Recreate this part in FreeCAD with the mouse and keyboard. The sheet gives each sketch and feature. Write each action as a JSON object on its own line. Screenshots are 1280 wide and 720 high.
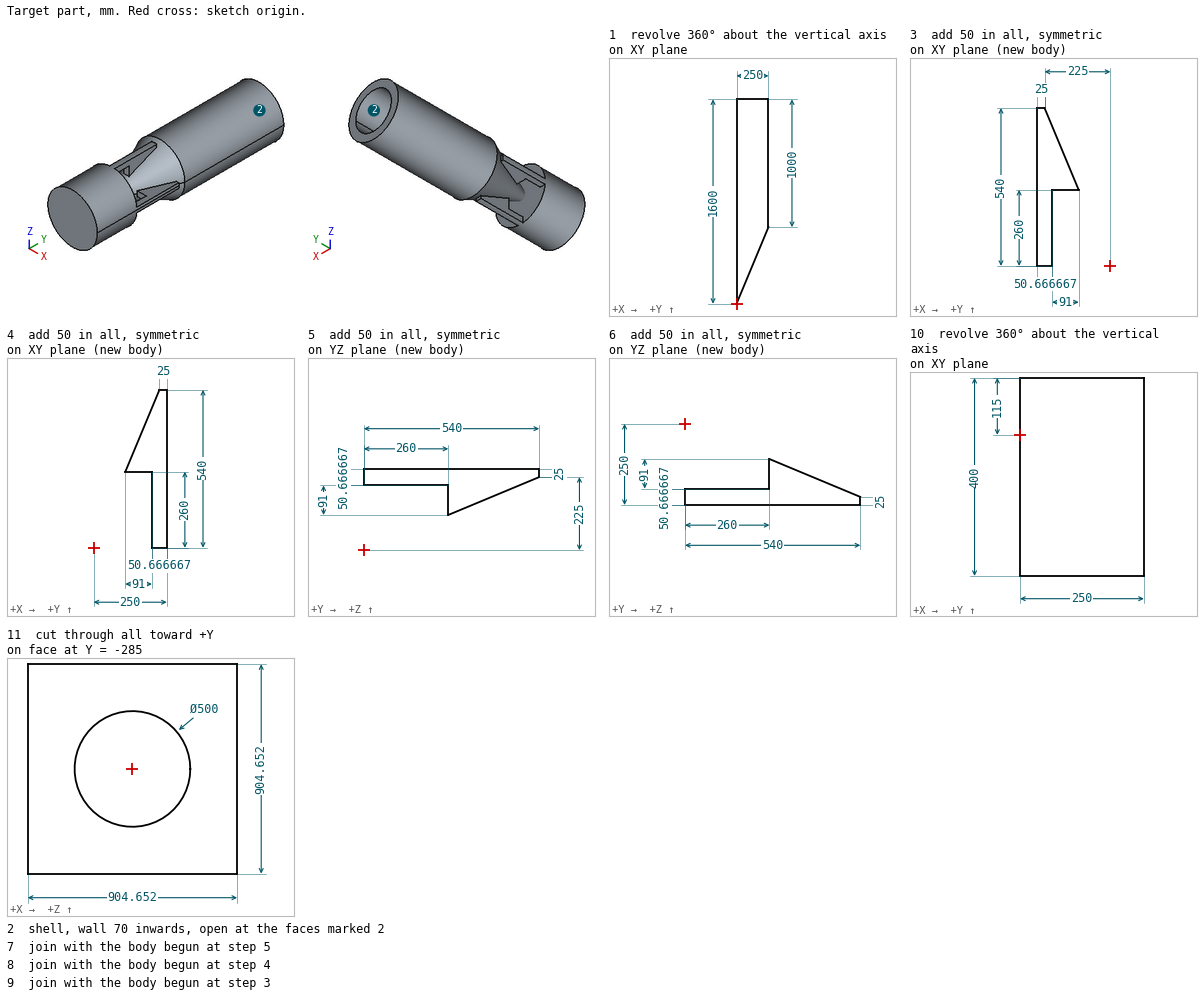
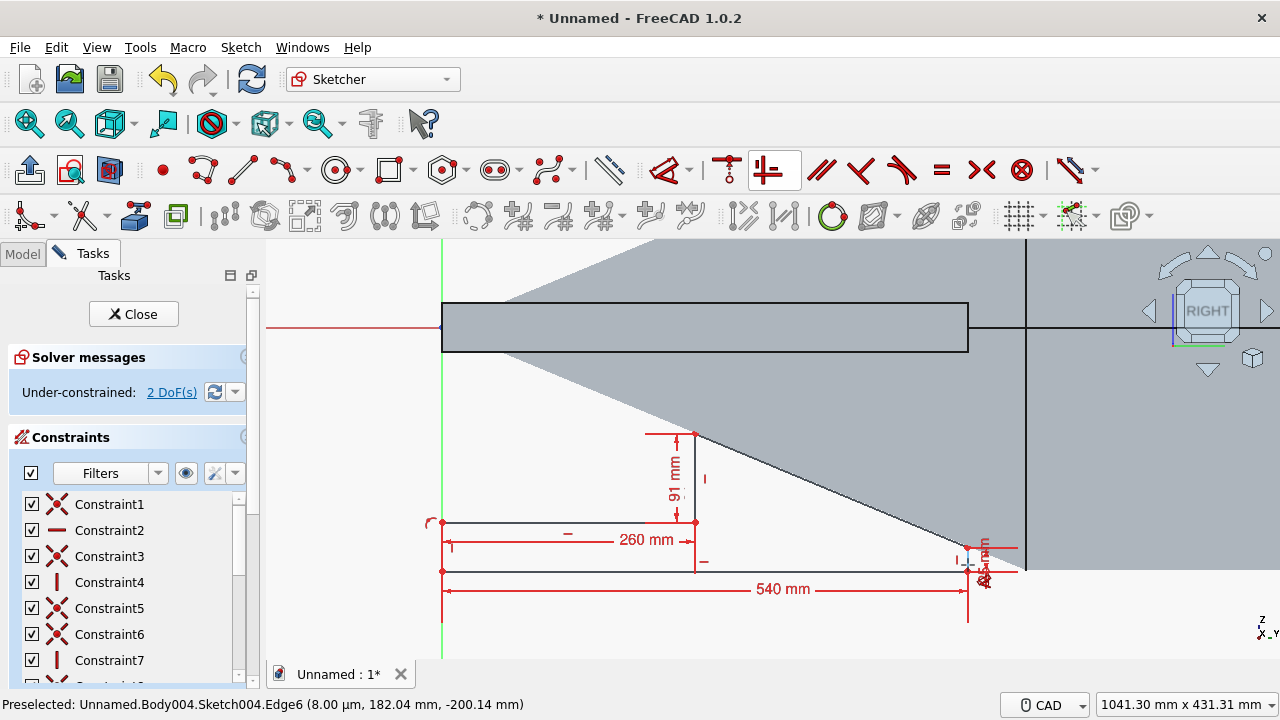
{"action": "left_click", "coordinate": [442, 572]}
{"action": "left_click", "coordinate": [408, 450]}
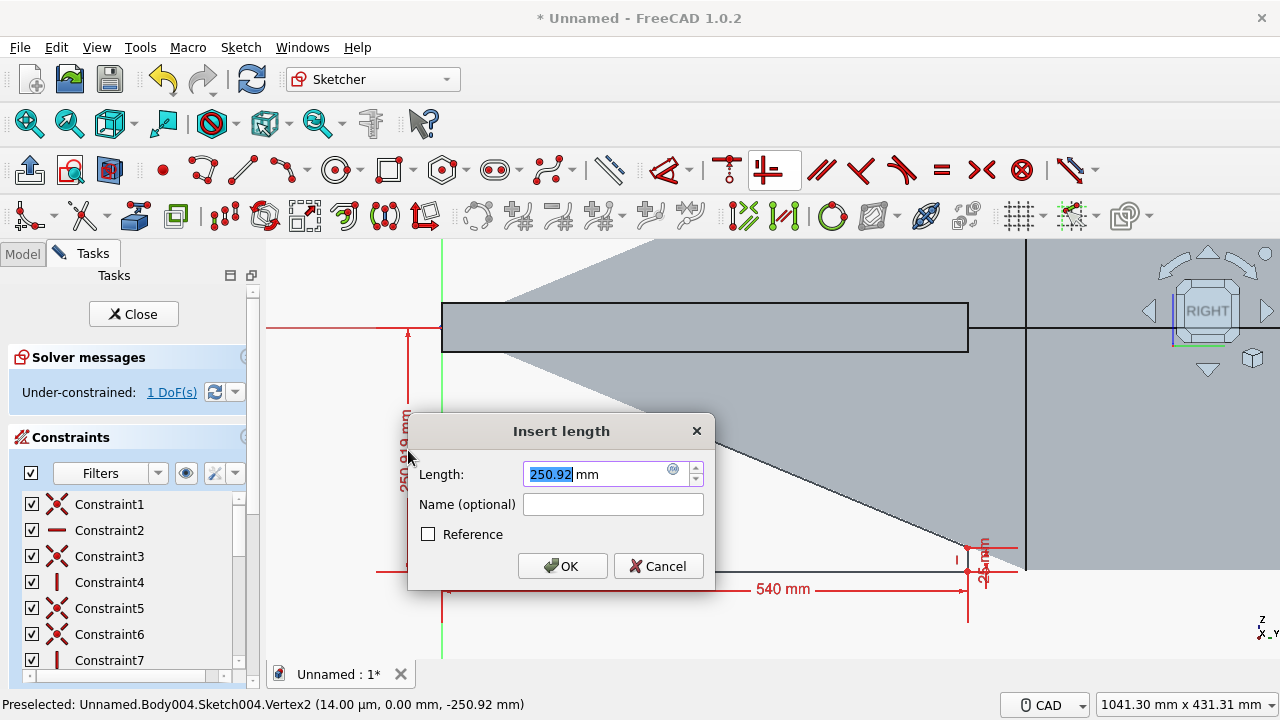
{"action": "type", "text": "250"}
{"action": "key", "text": "Return"}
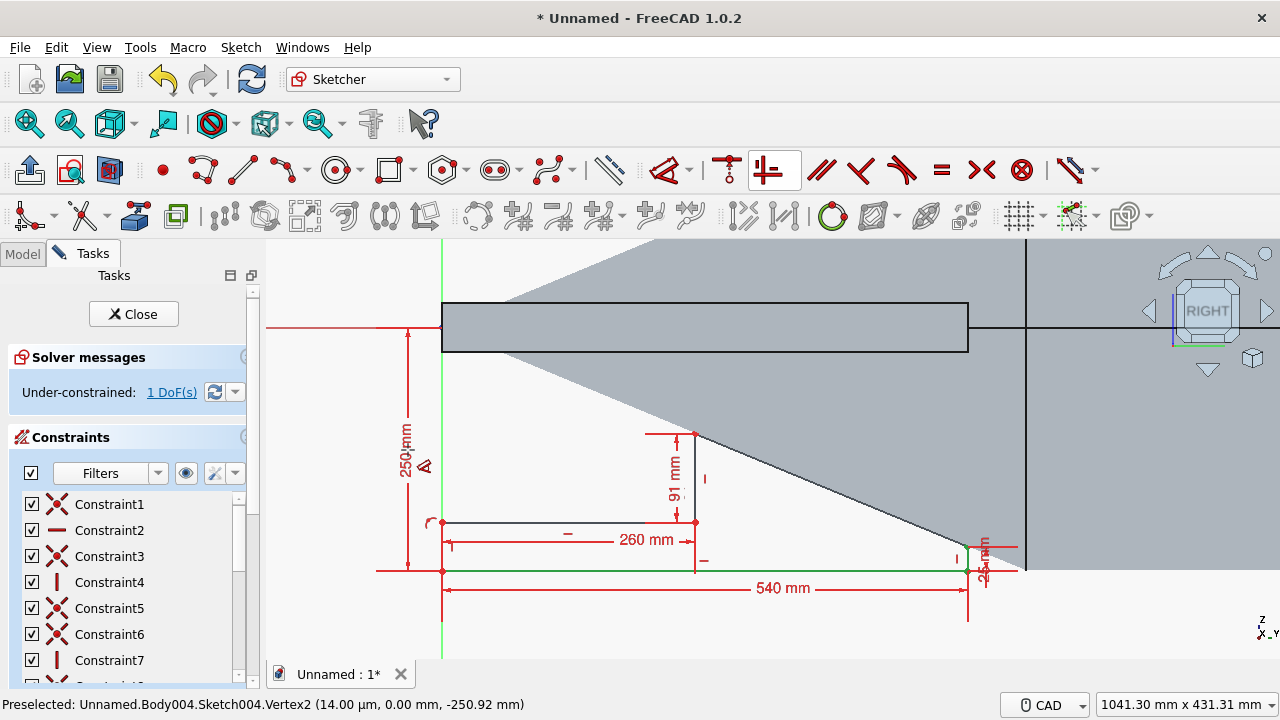
{"action": "left_click", "coordinate": [442, 537]}
{"action": "left_click", "coordinate": [408, 547]}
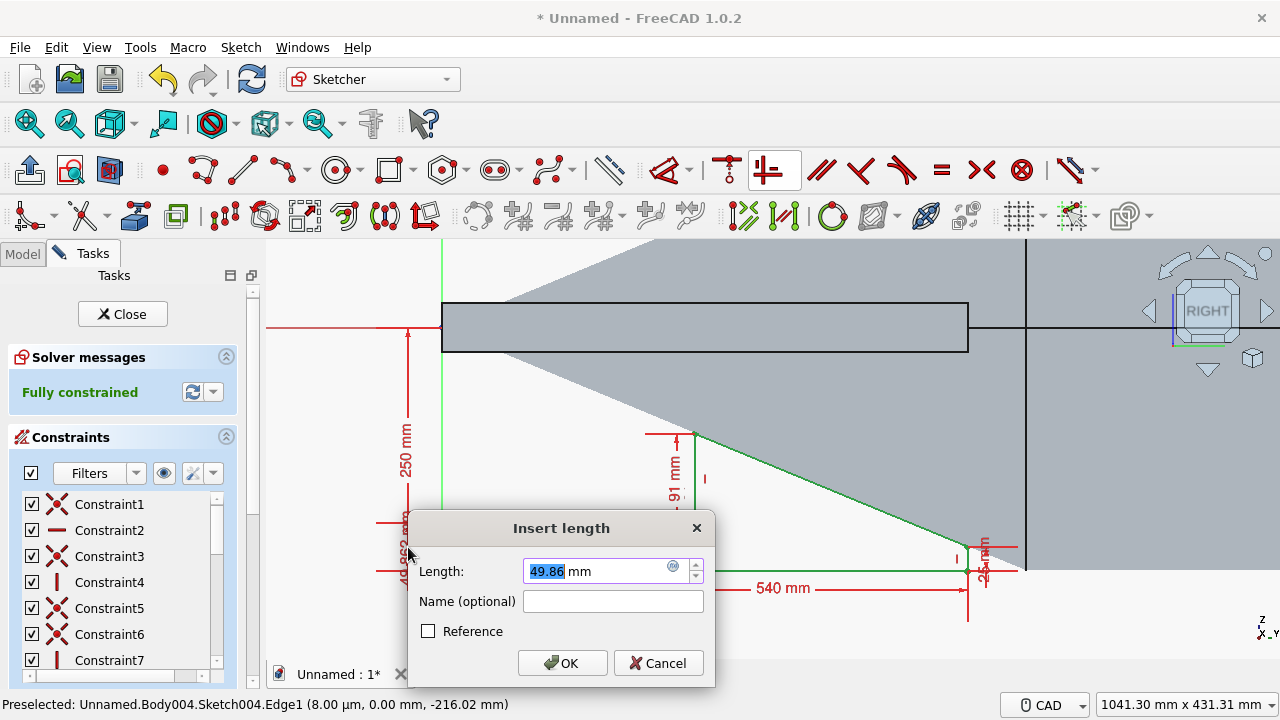
{"action": "type", "text": "50.666667"}
{"action": "key", "text": "Return"}
{"action": "key", "text": "Escape"}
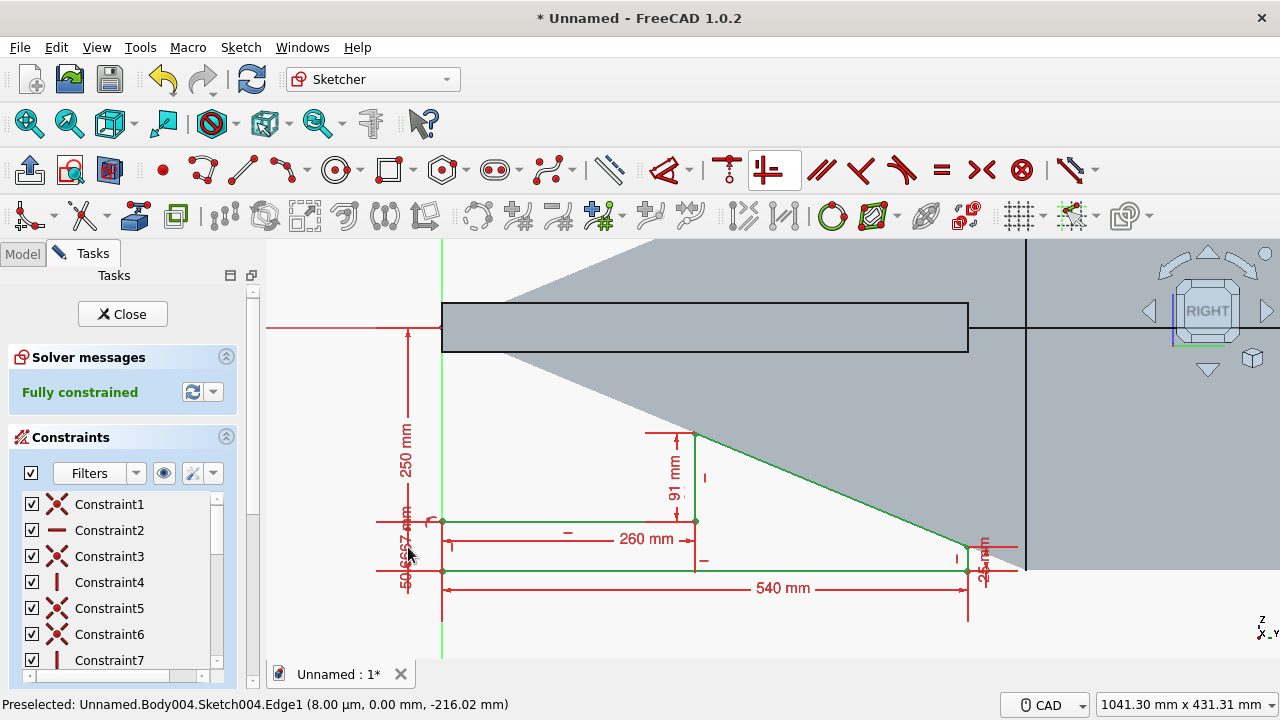
{"action": "left_click", "coordinate": [123, 314]}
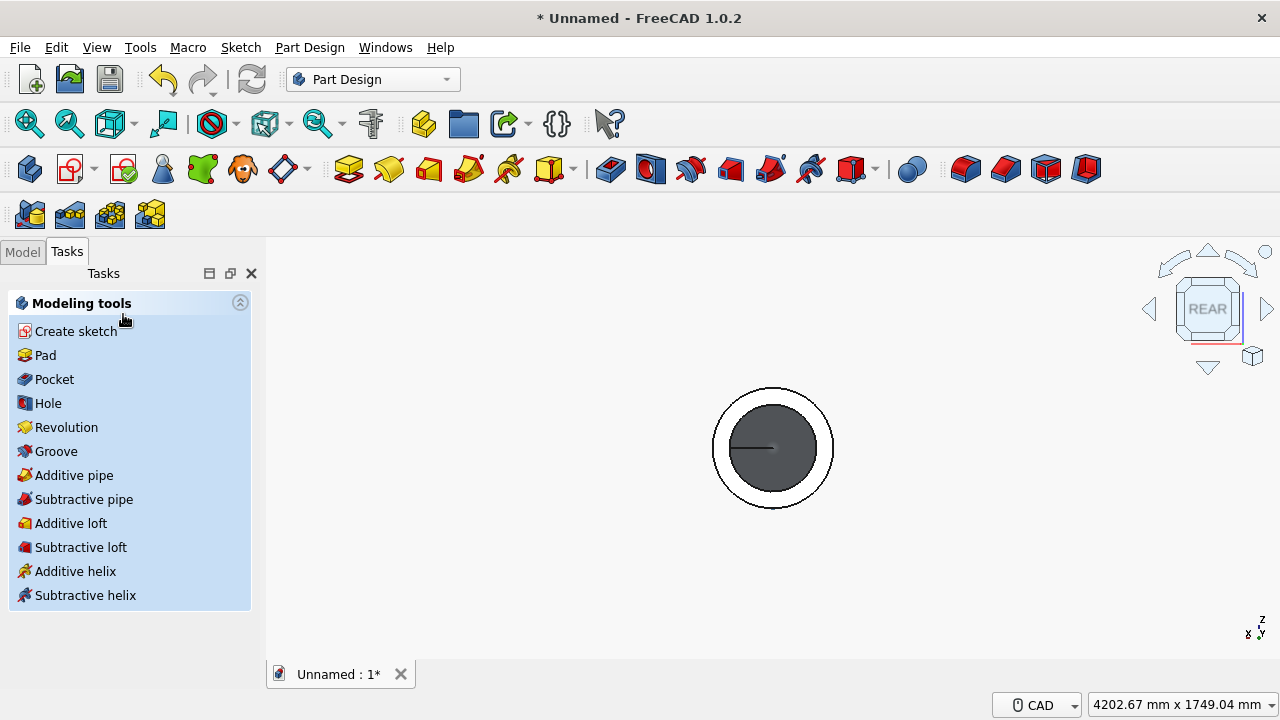
{"action": "left_click", "coordinate": [350, 170]}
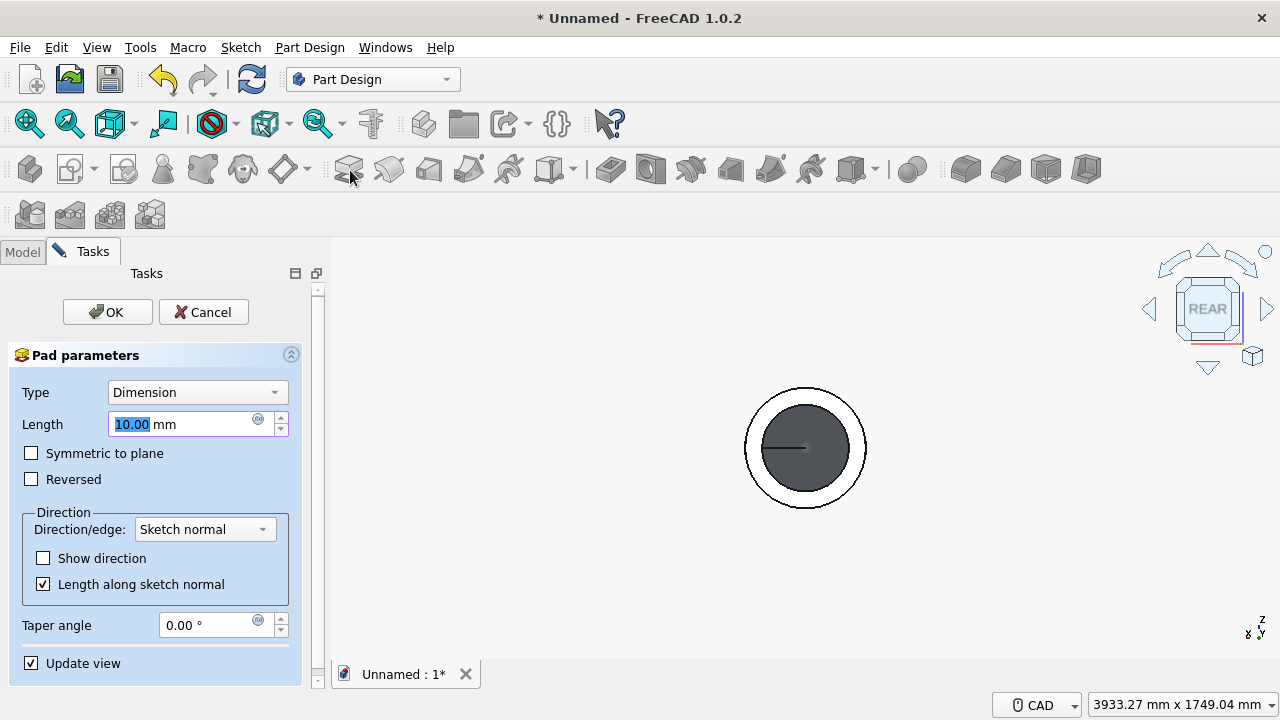
{"action": "type", "text": "50"}
{"action": "key", "text": "Tab"}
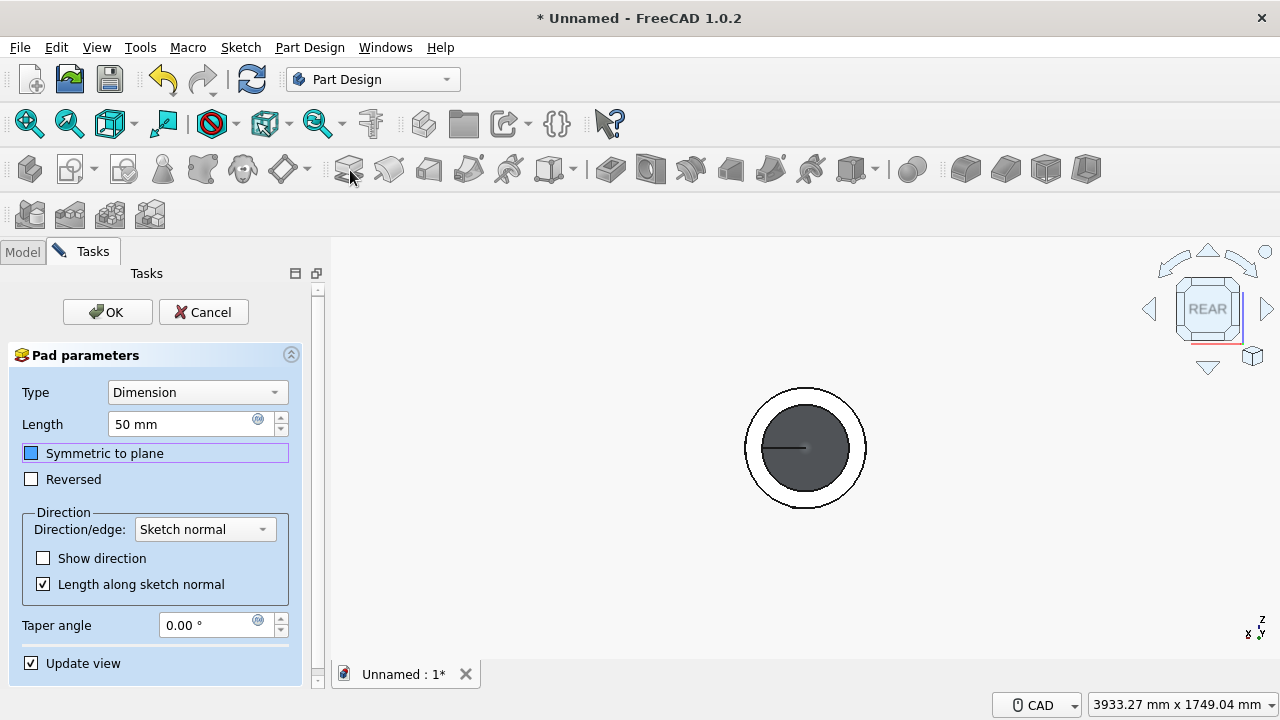
{"action": "left_click", "coordinate": [30, 453]}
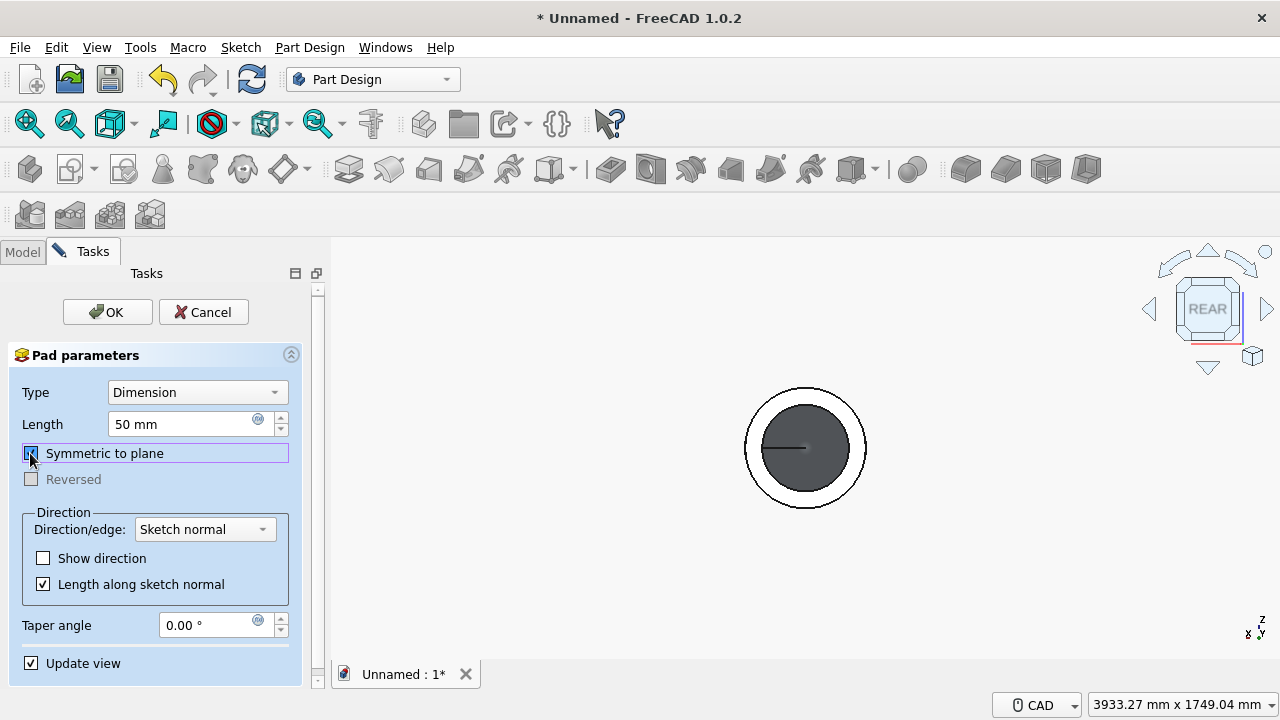
{"action": "left_click", "coordinate": [108, 312]}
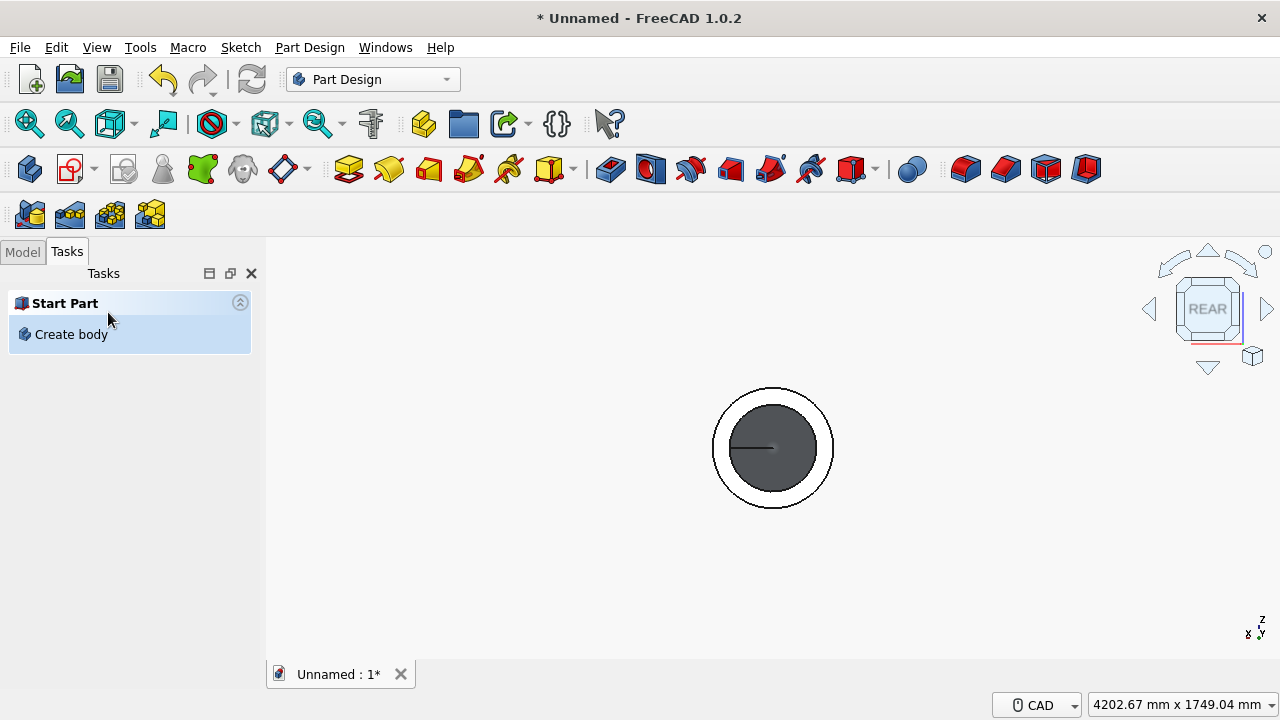
{"action": "left_click", "coordinate": [30, 124]}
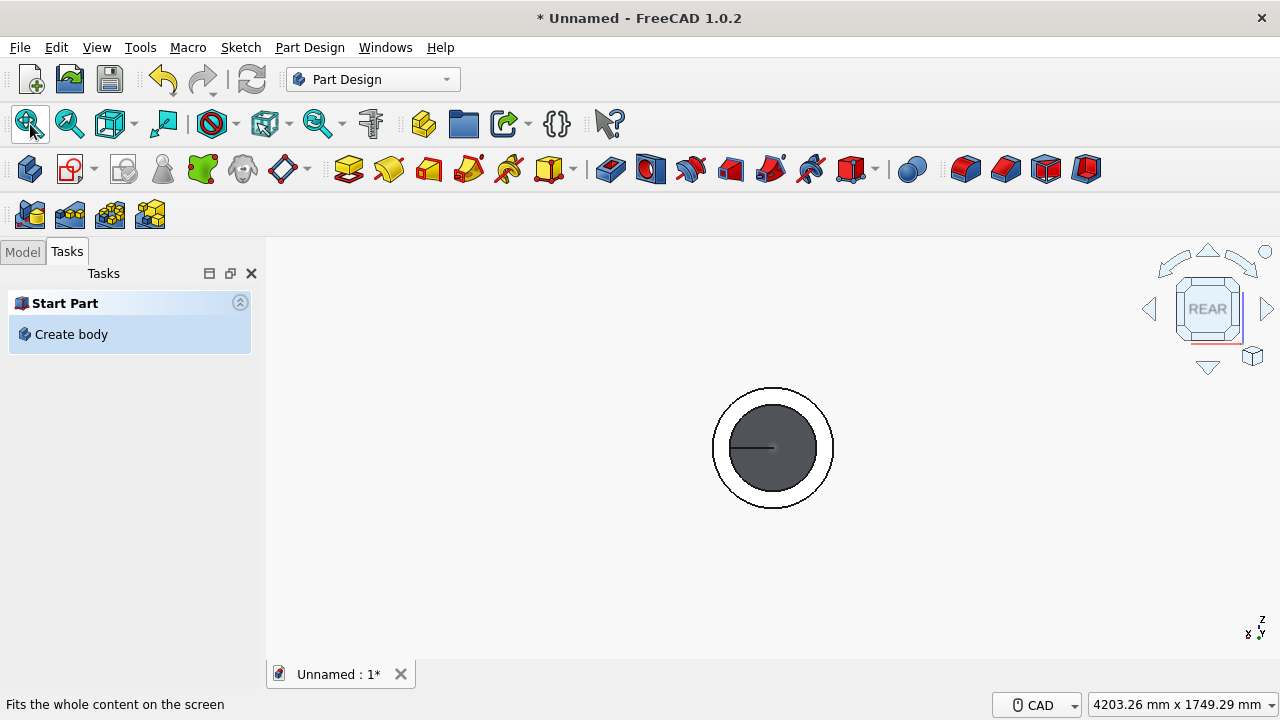
{"action": "left_click", "coordinate": [23, 251]}